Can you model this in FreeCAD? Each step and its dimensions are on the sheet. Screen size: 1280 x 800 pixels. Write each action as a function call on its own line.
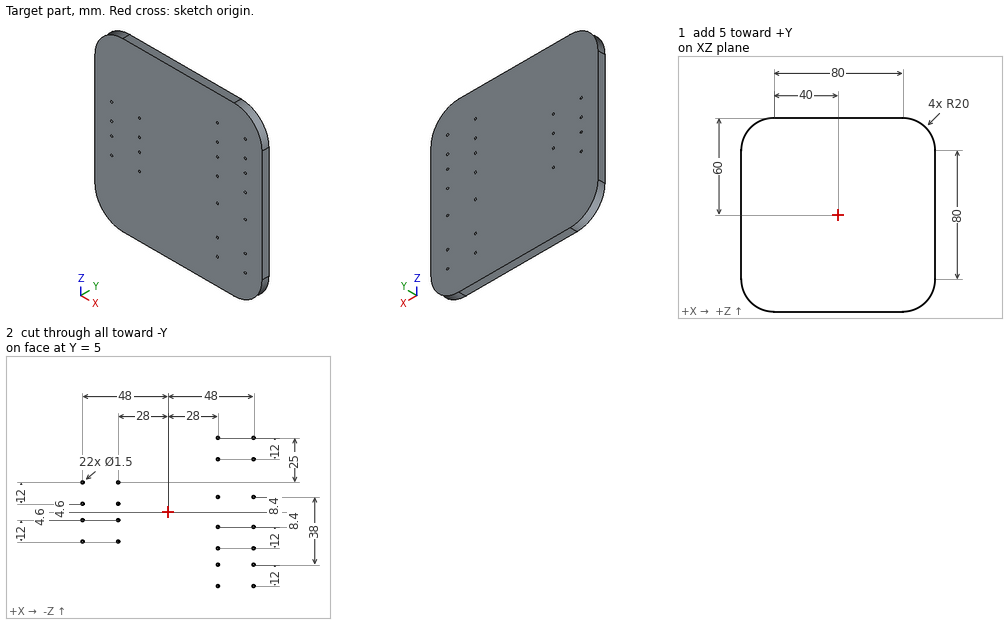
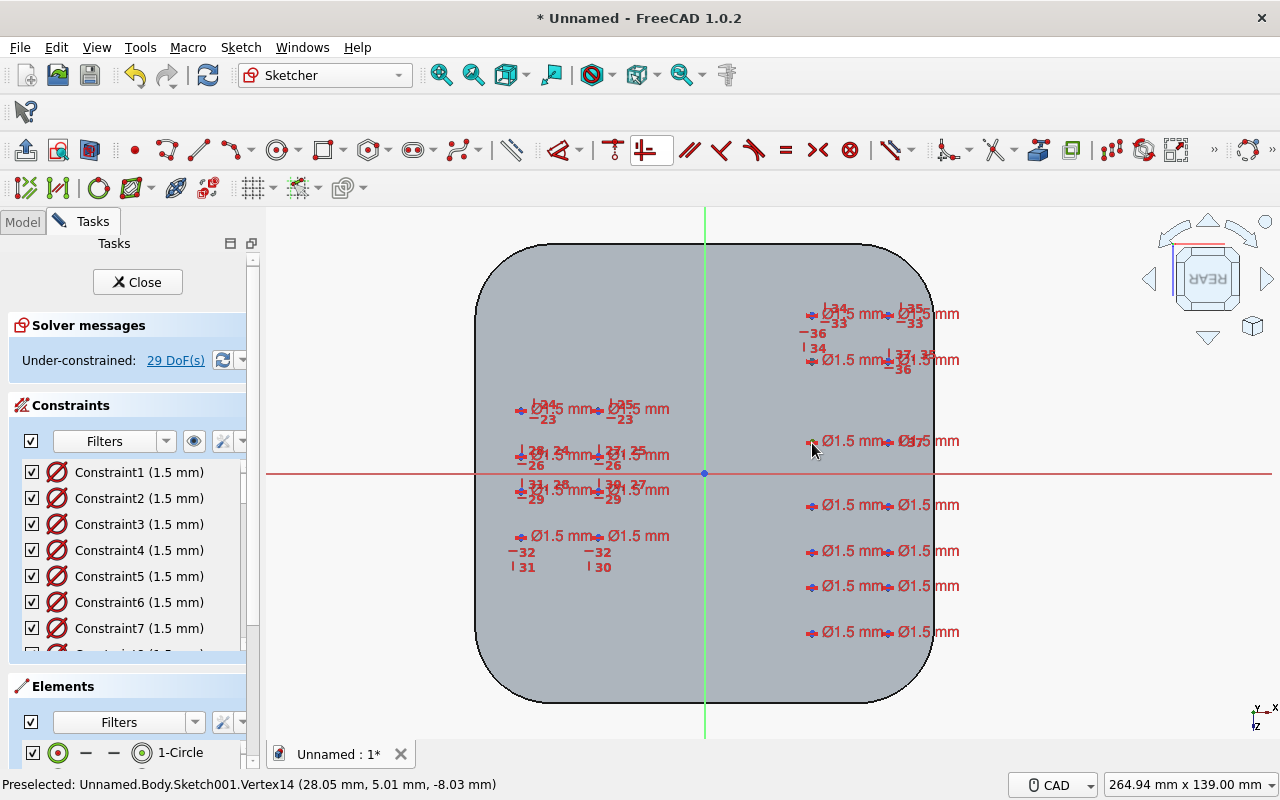
key(v)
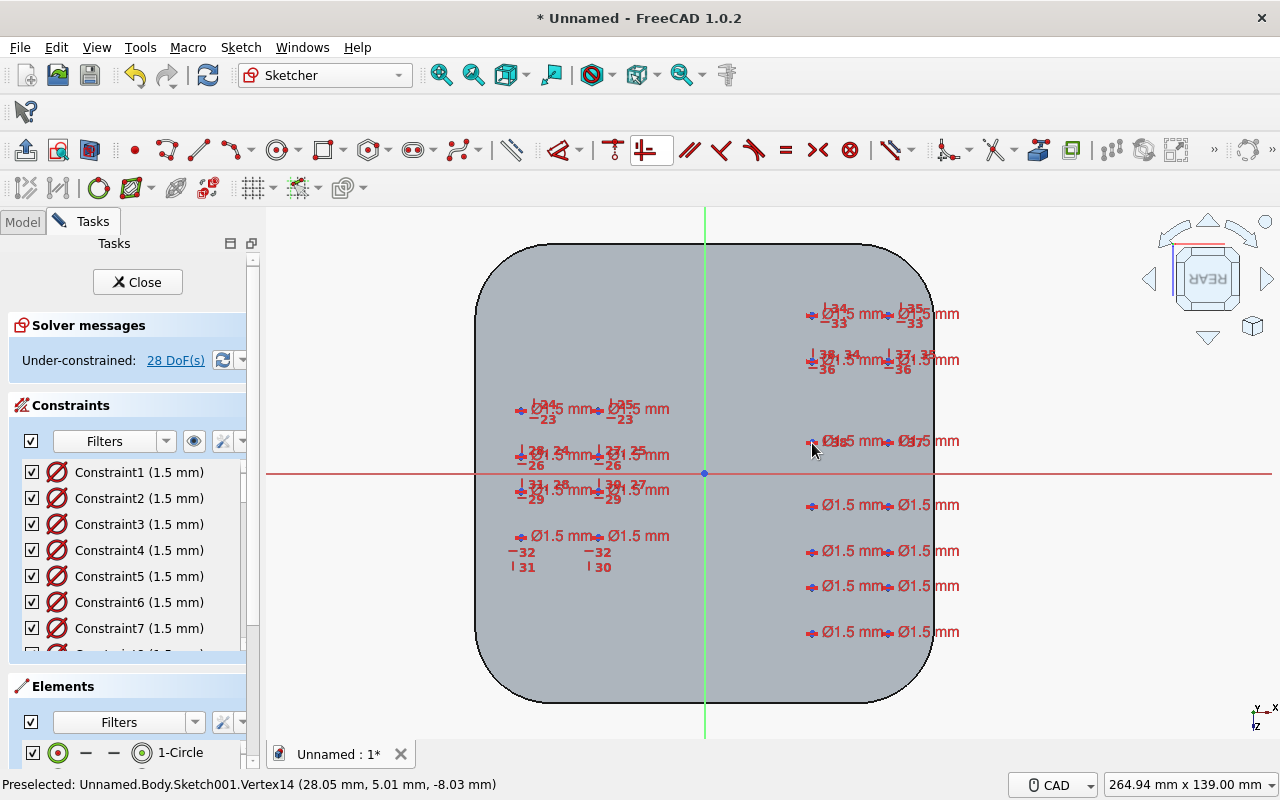
click(888, 443)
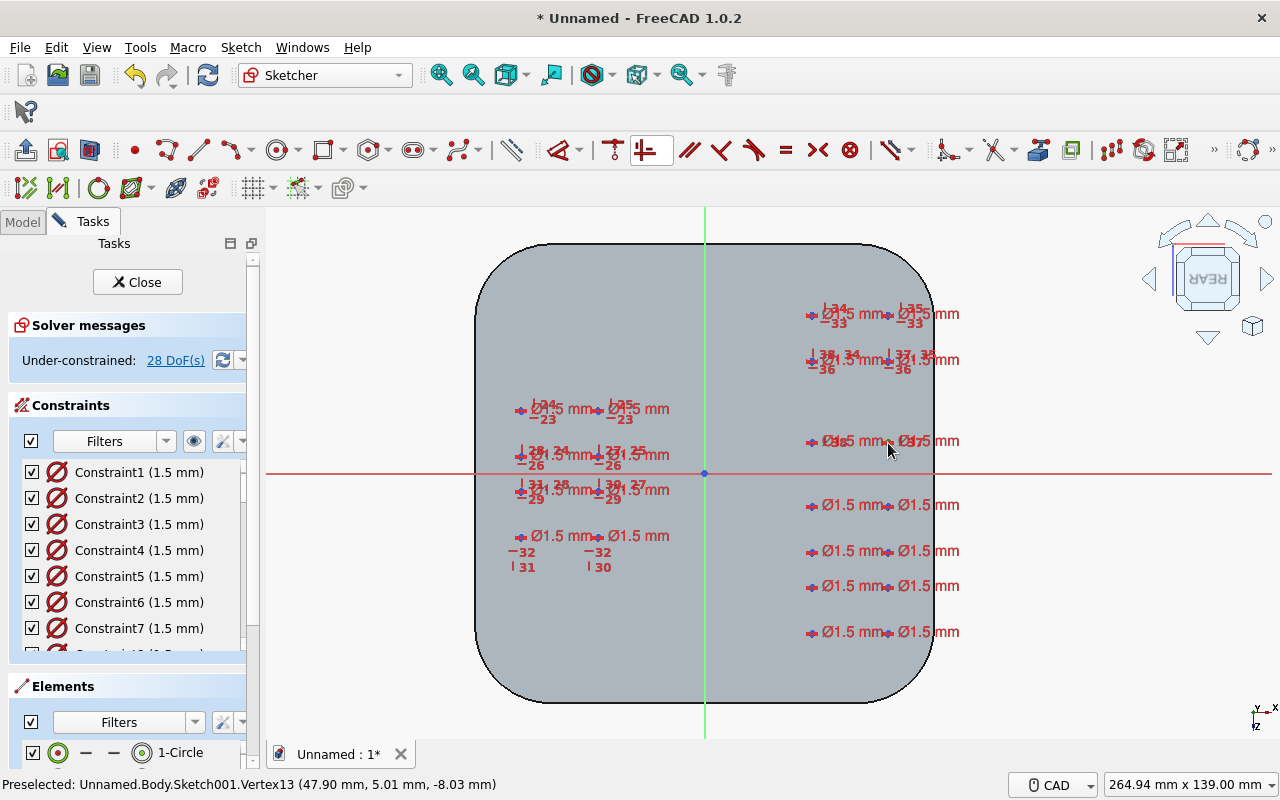
click(812, 443)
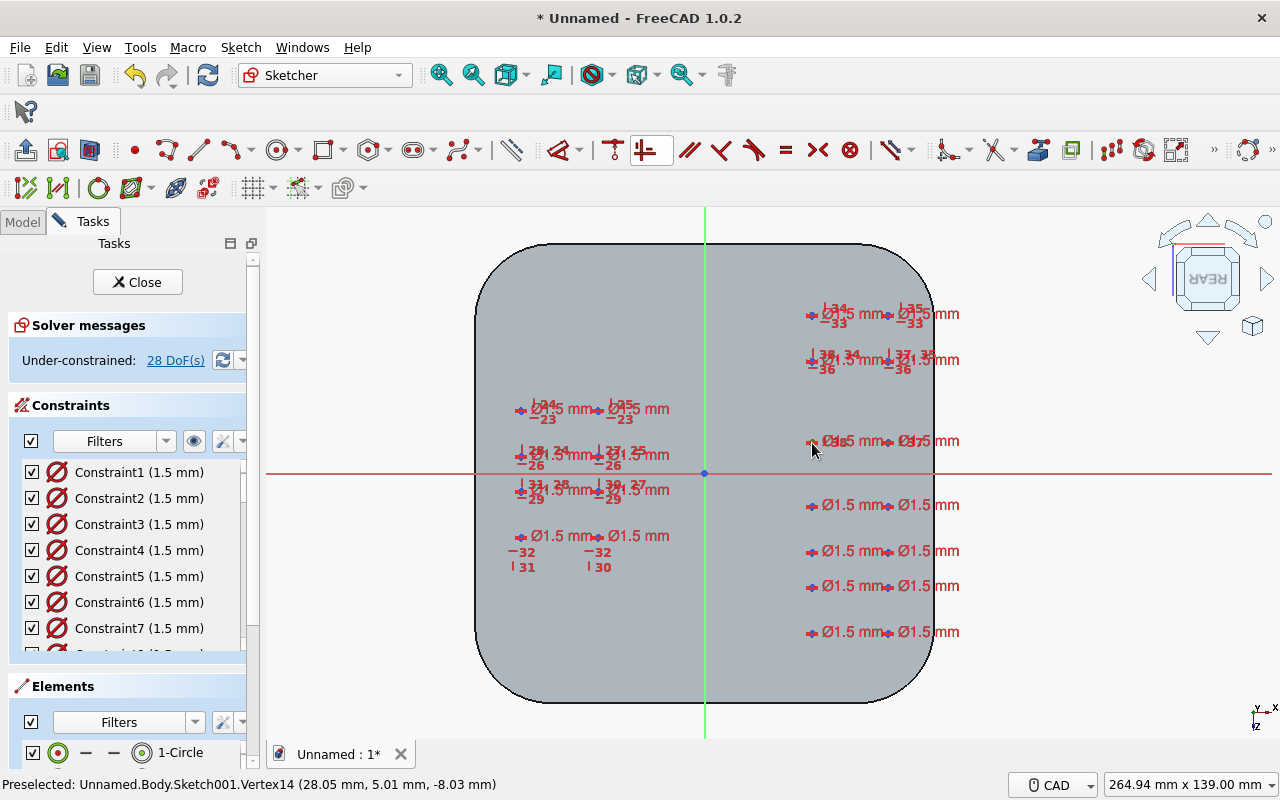
click(668, 150)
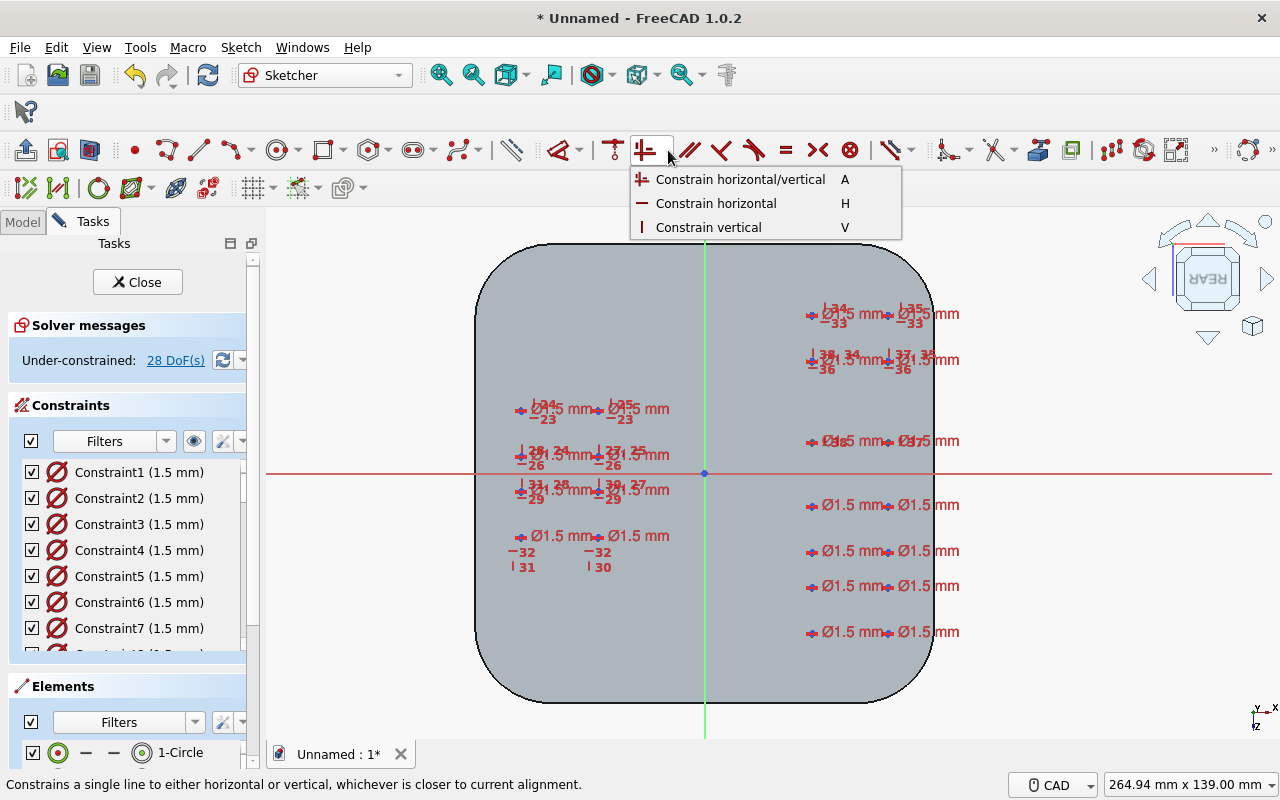
click(766, 203)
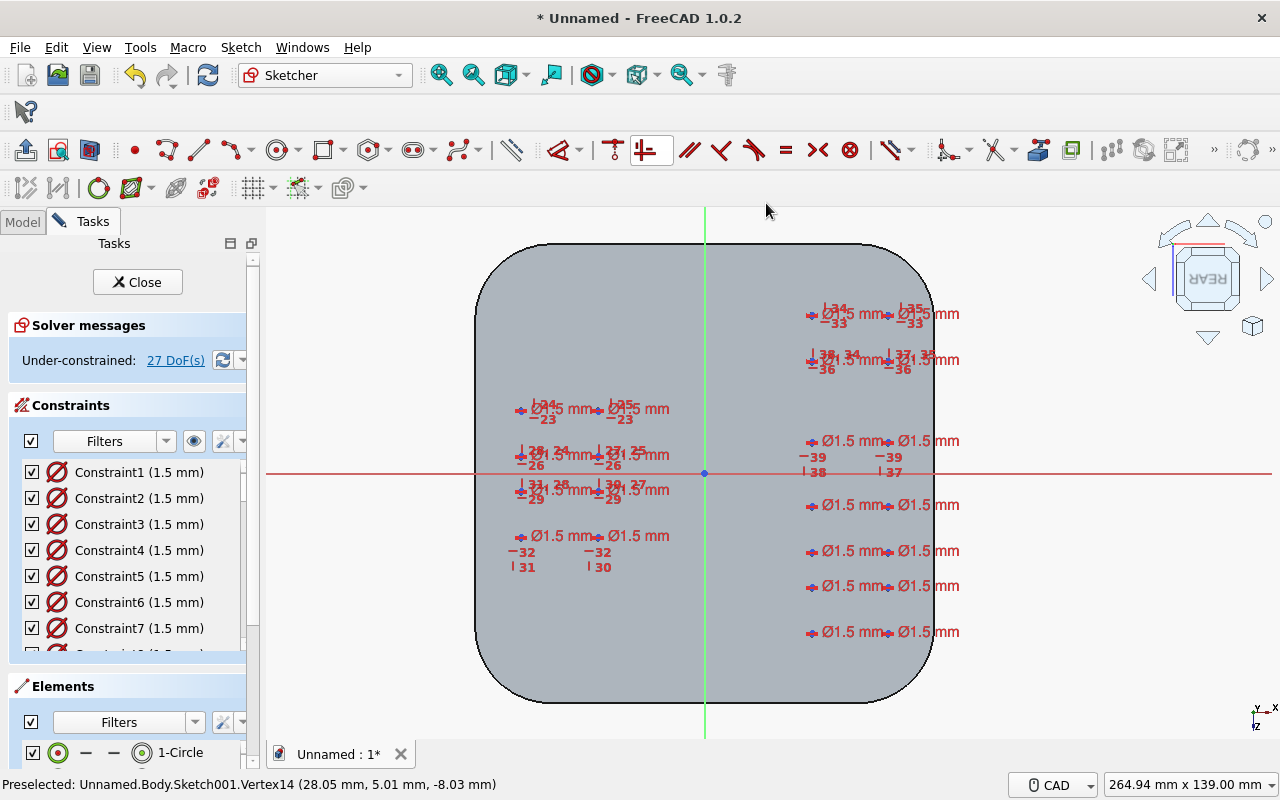
click(812, 443)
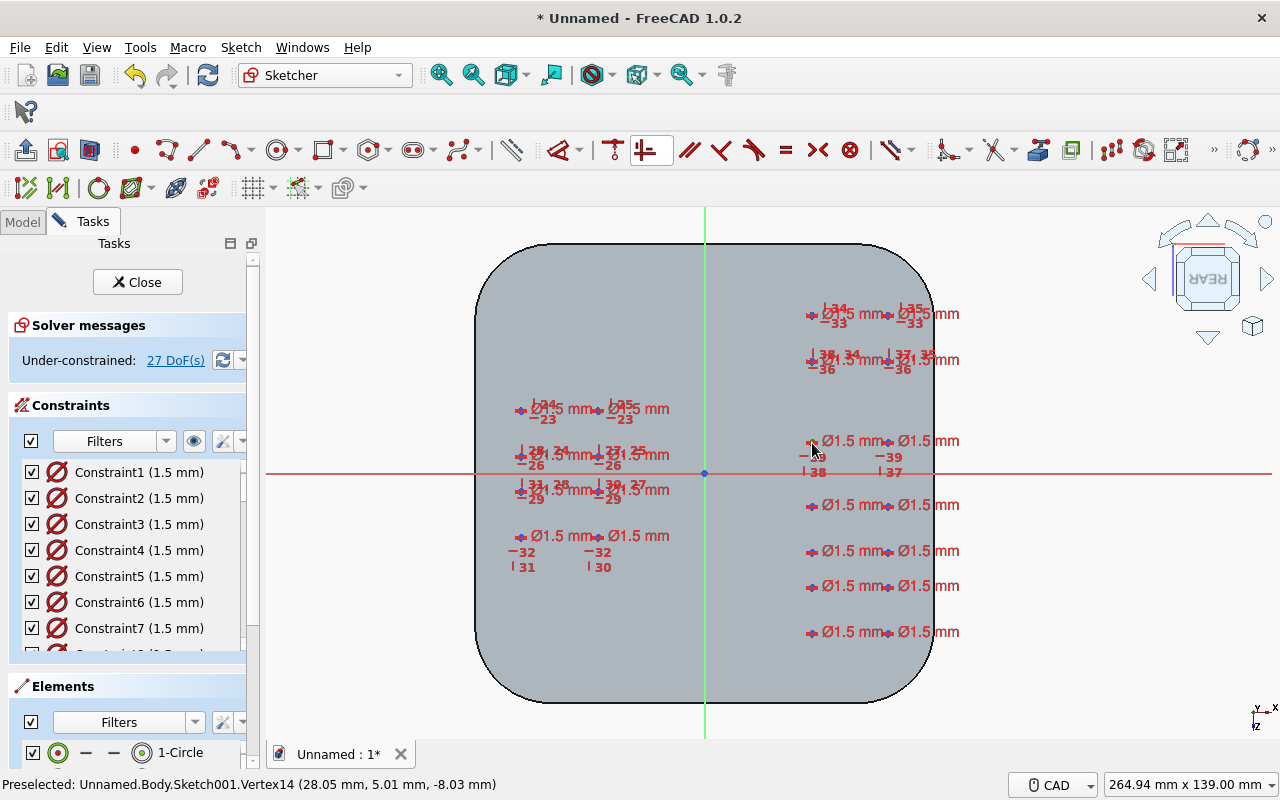
click(812, 507)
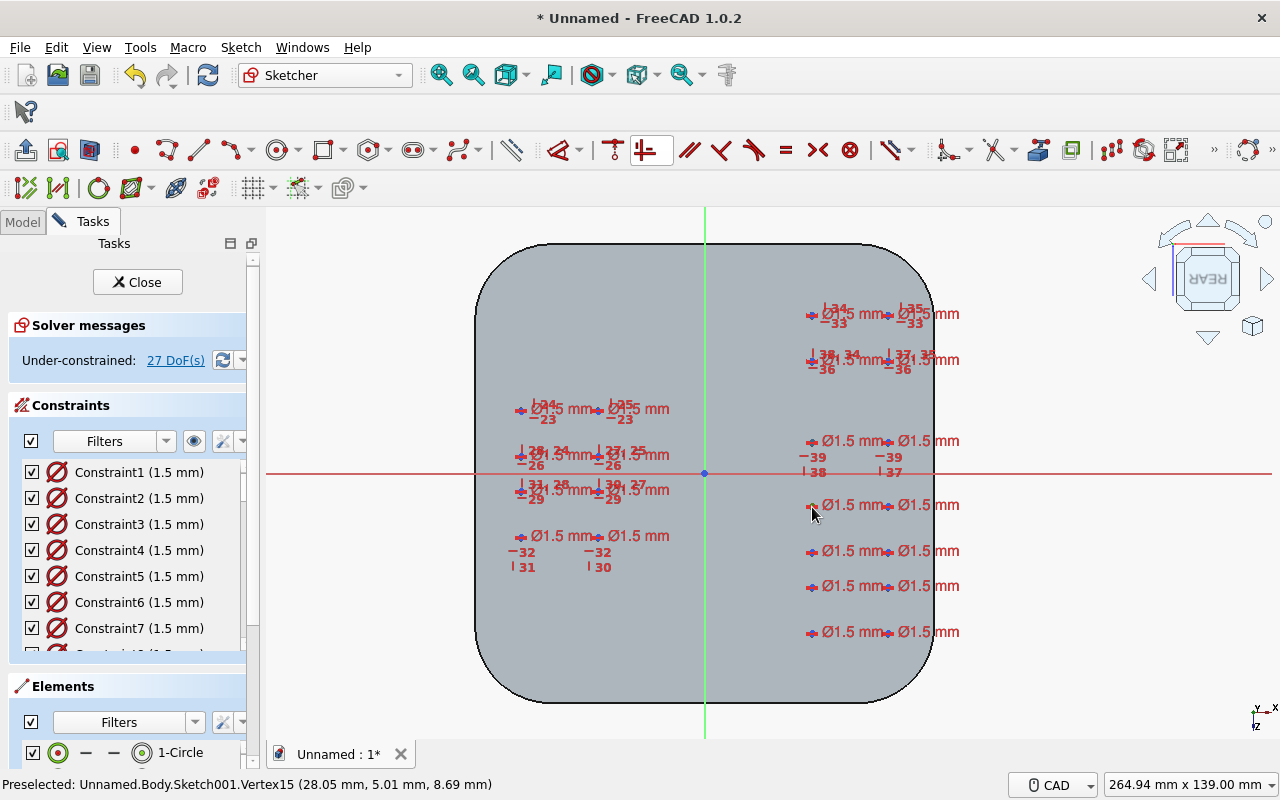
click(668, 150)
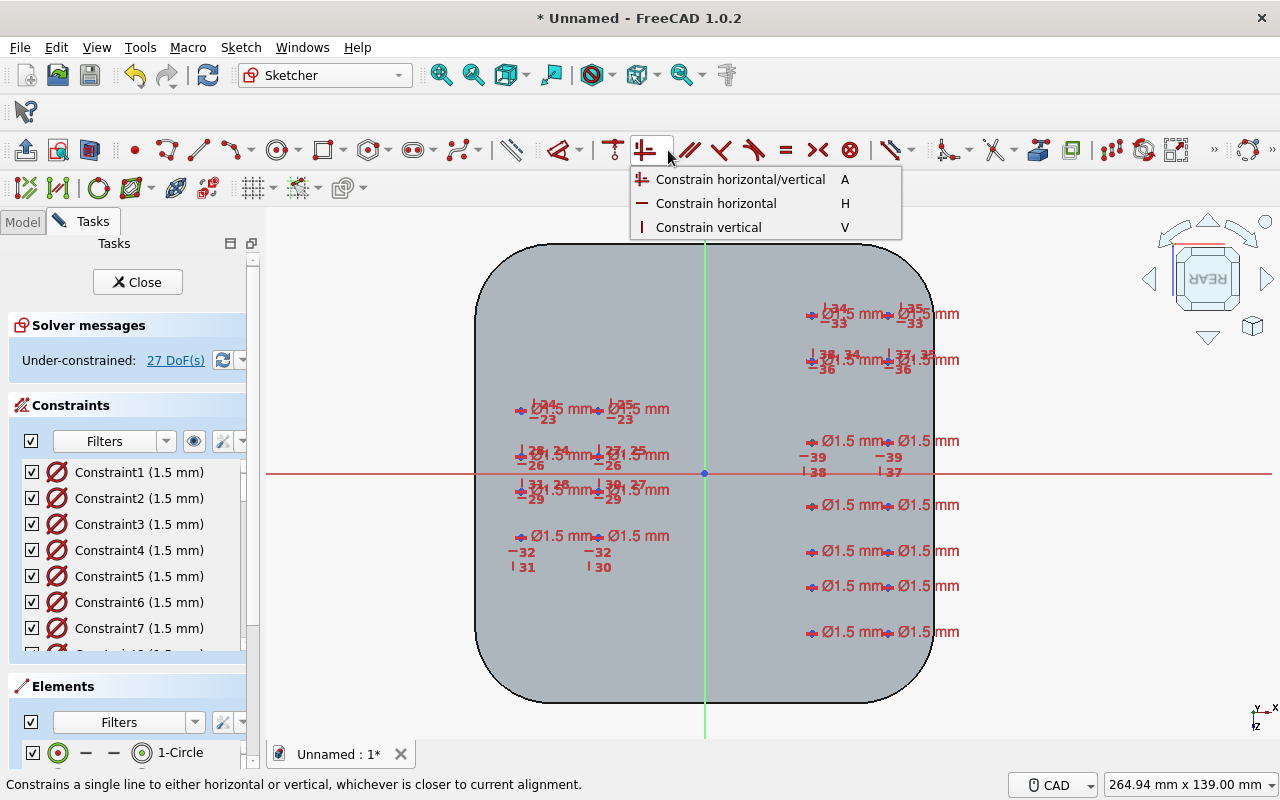
click(766, 227)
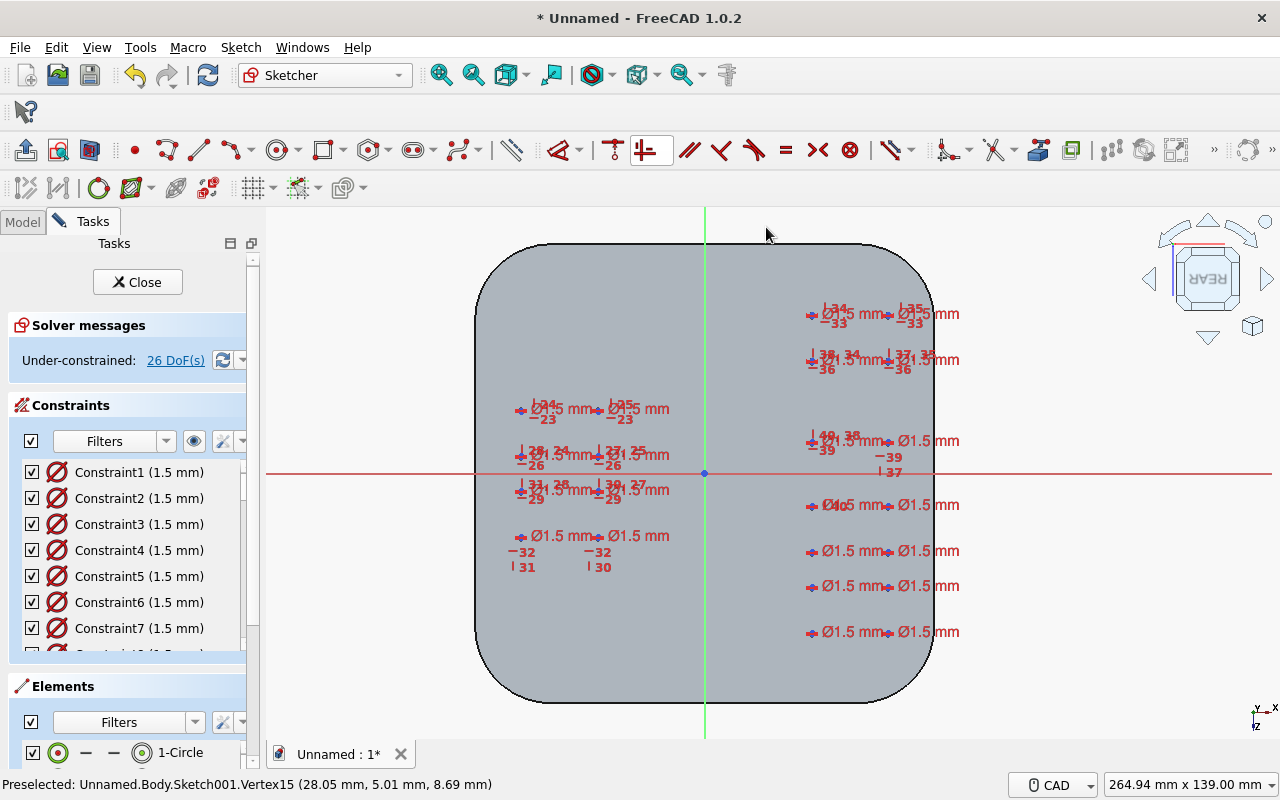
click(888, 443)